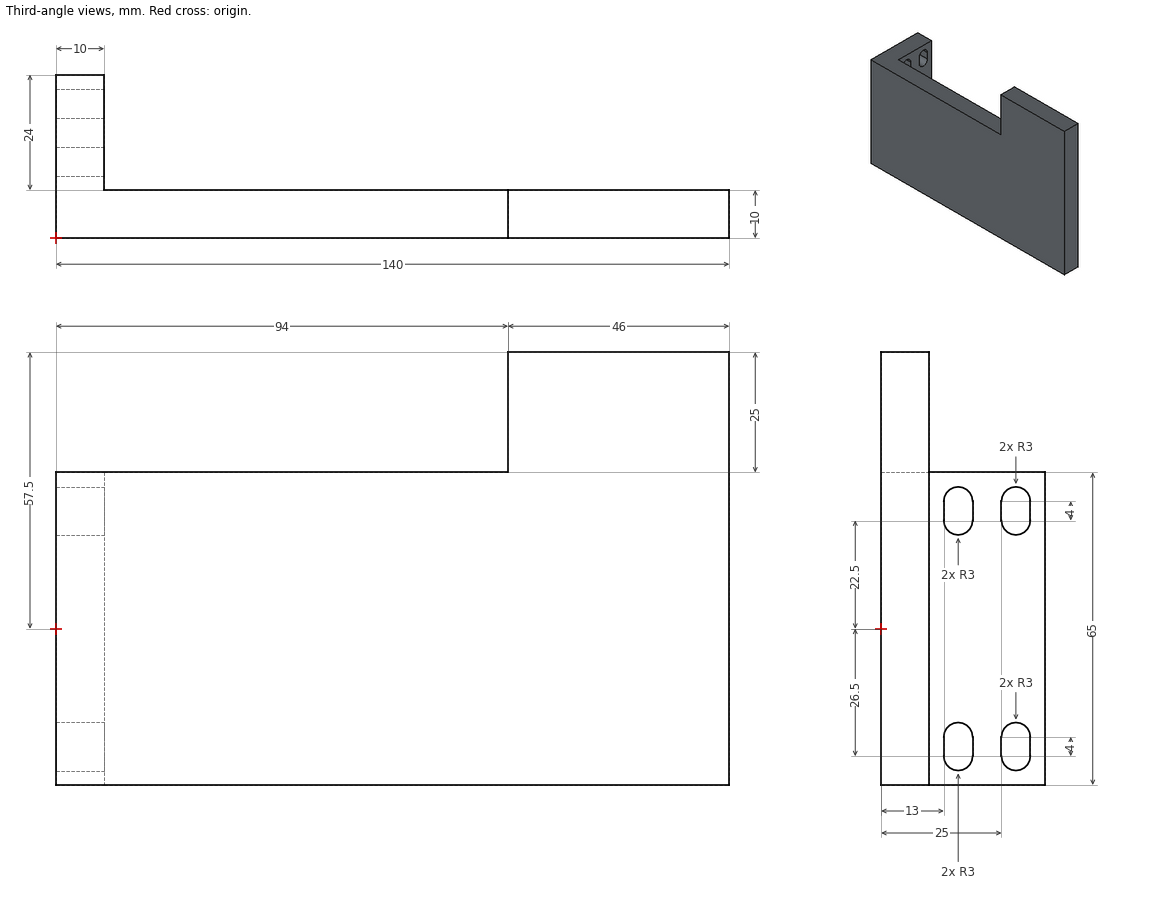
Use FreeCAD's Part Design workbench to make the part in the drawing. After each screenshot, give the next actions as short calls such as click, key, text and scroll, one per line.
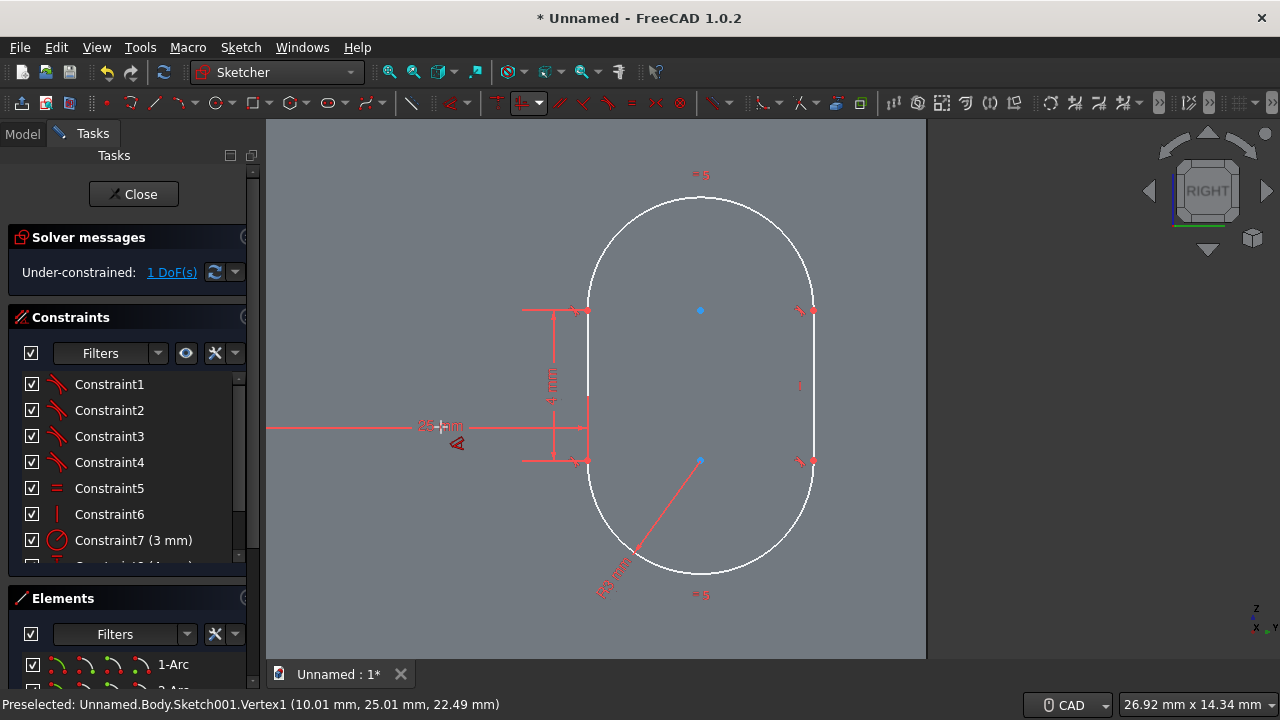
click(588, 461)
click(622, 507)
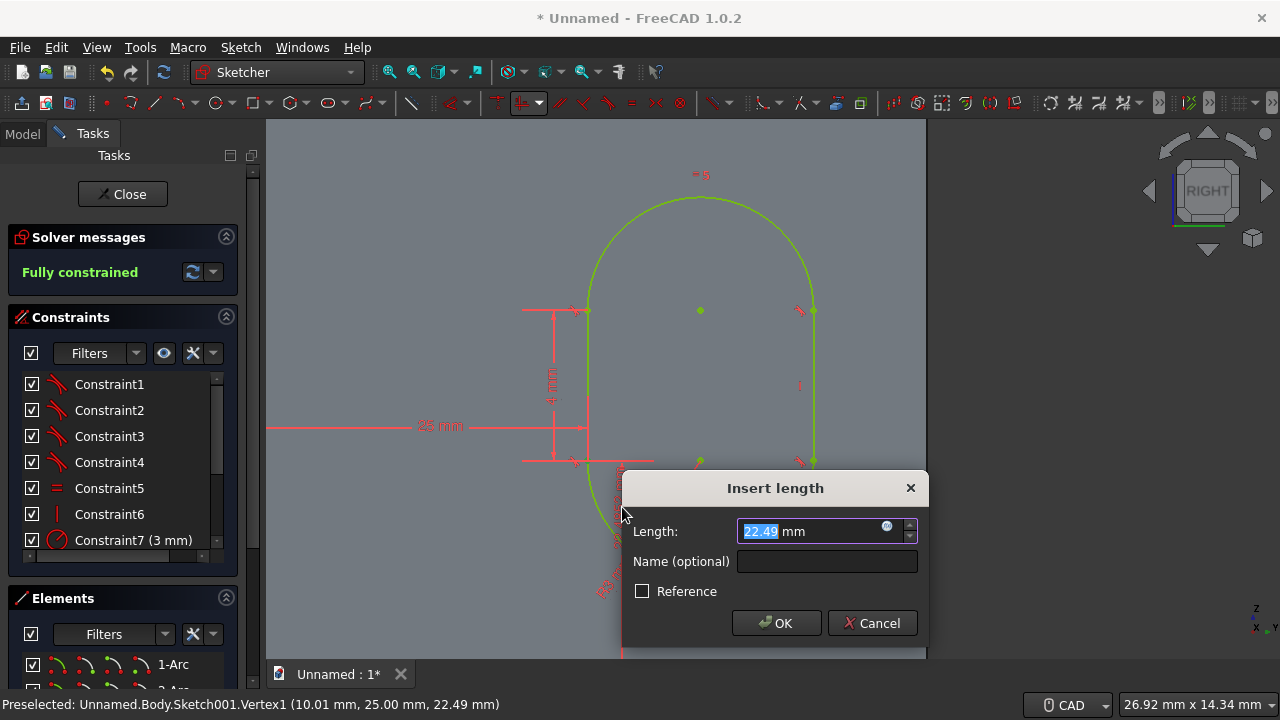
text(22.5)
key(Return)
key(Escape)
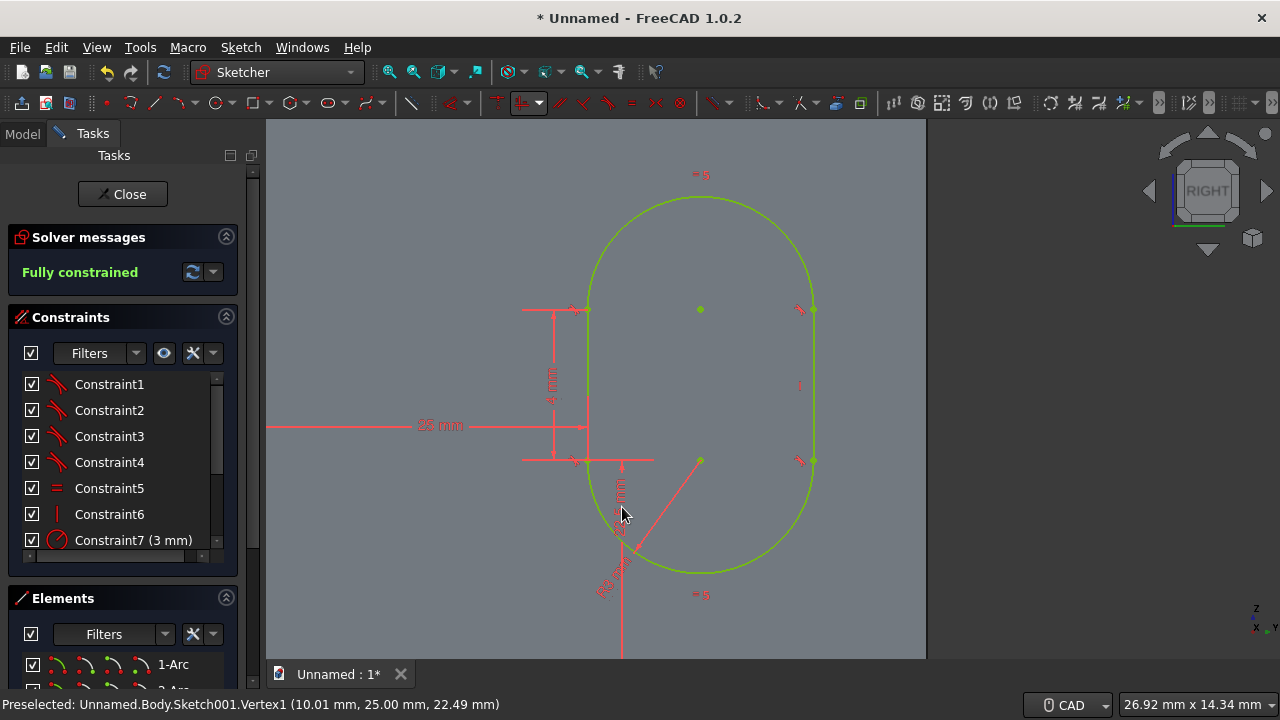
click(123, 194)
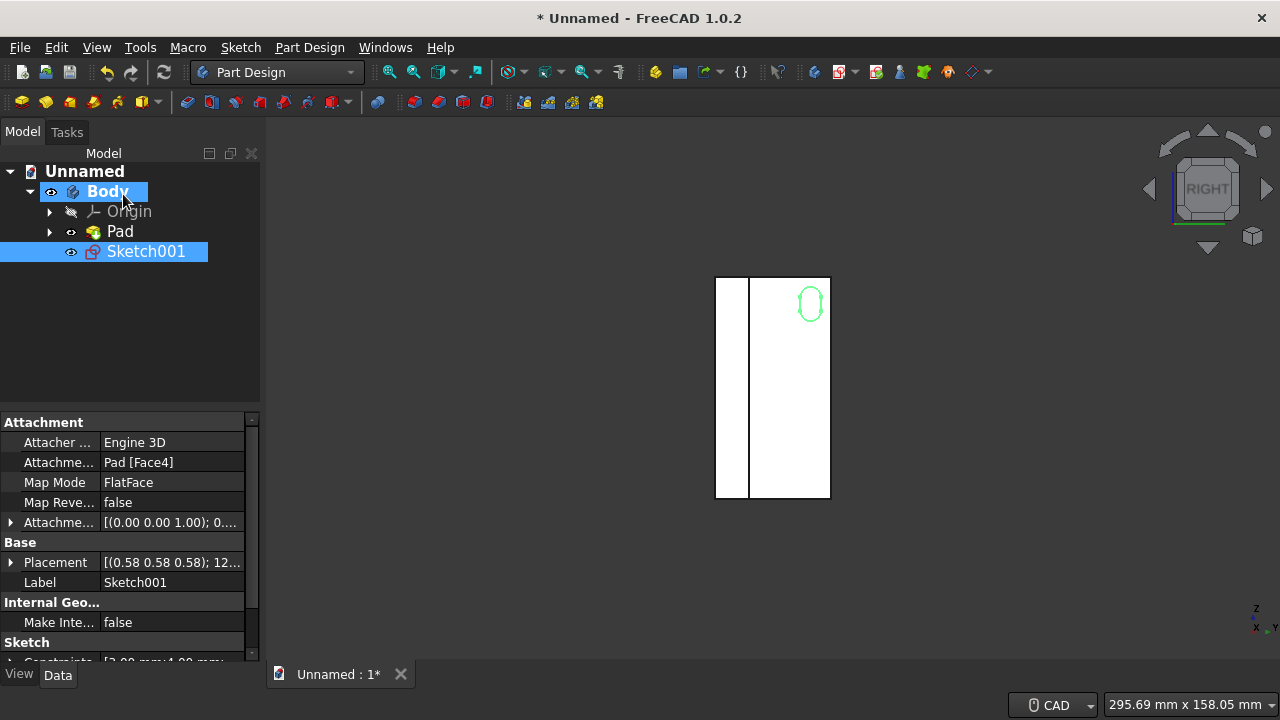
click(188, 102)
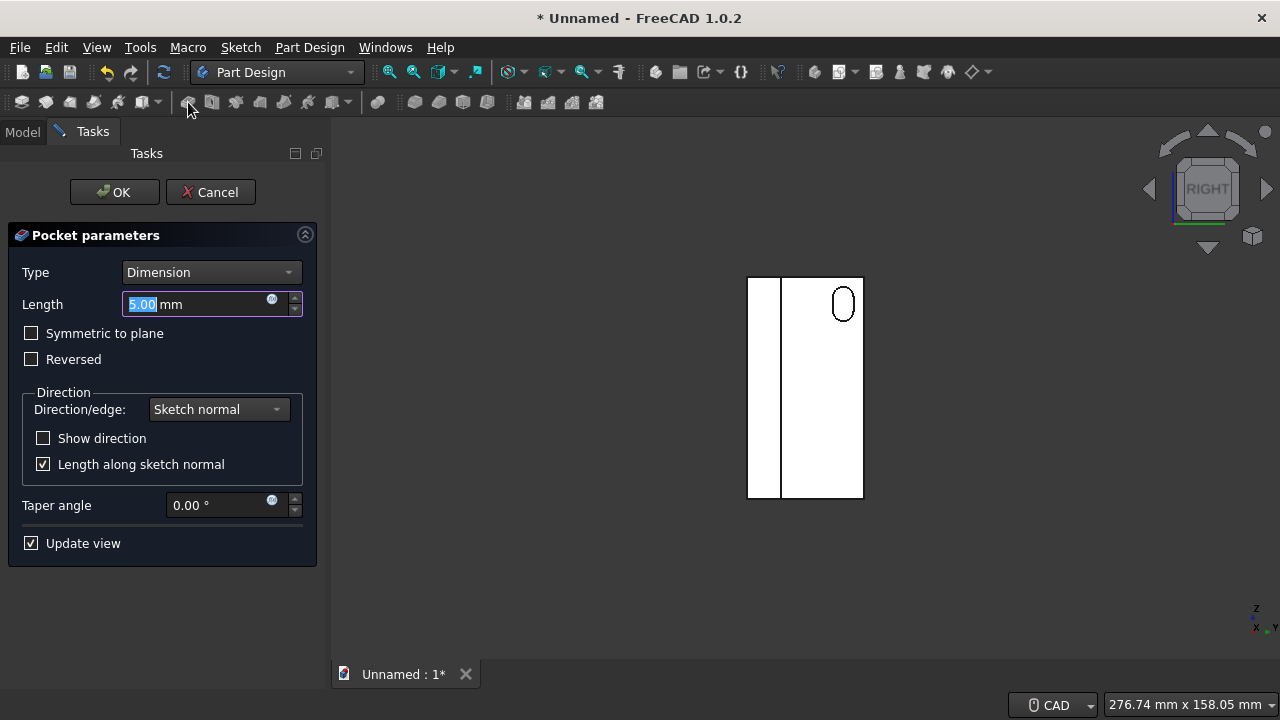
click(212, 272)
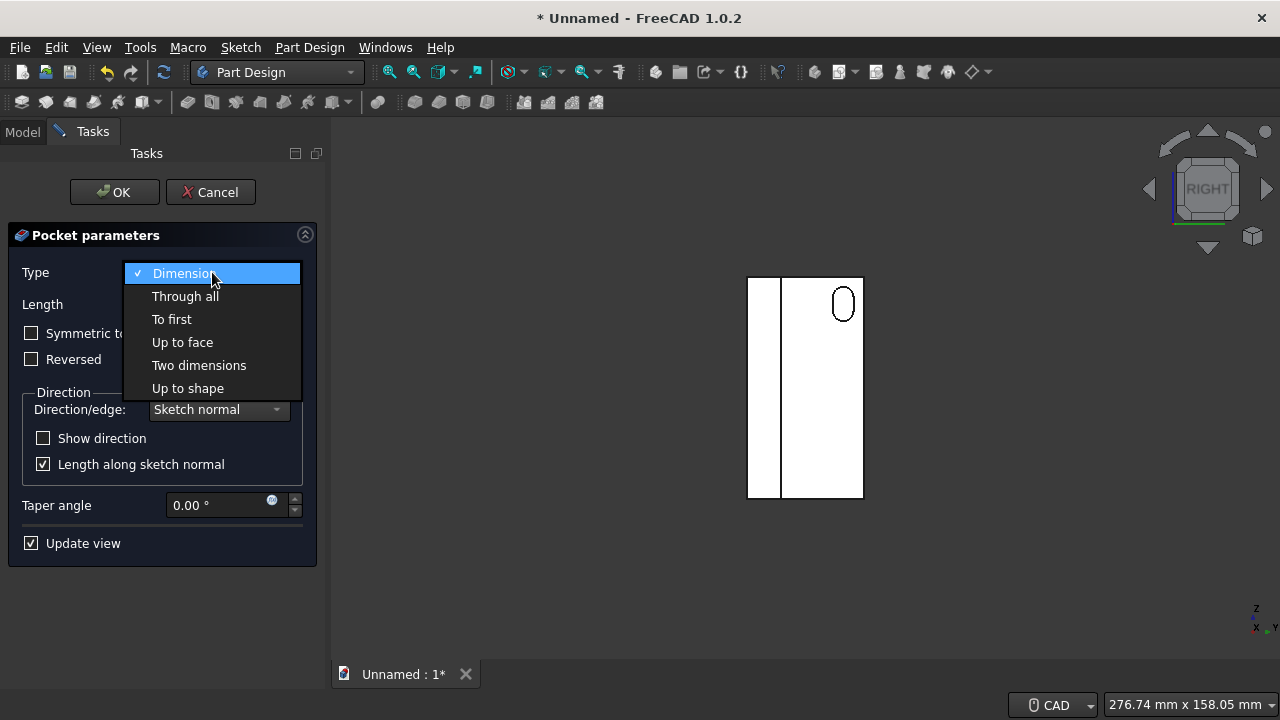
click(212, 320)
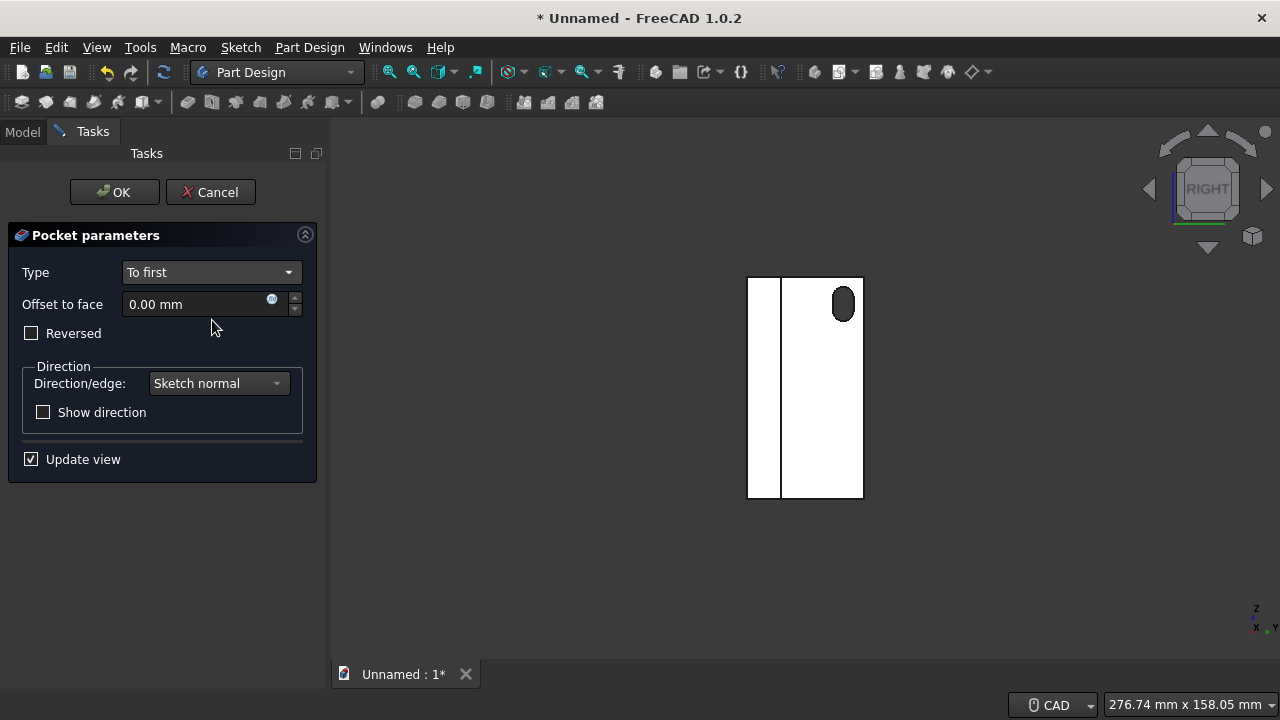
click(115, 192)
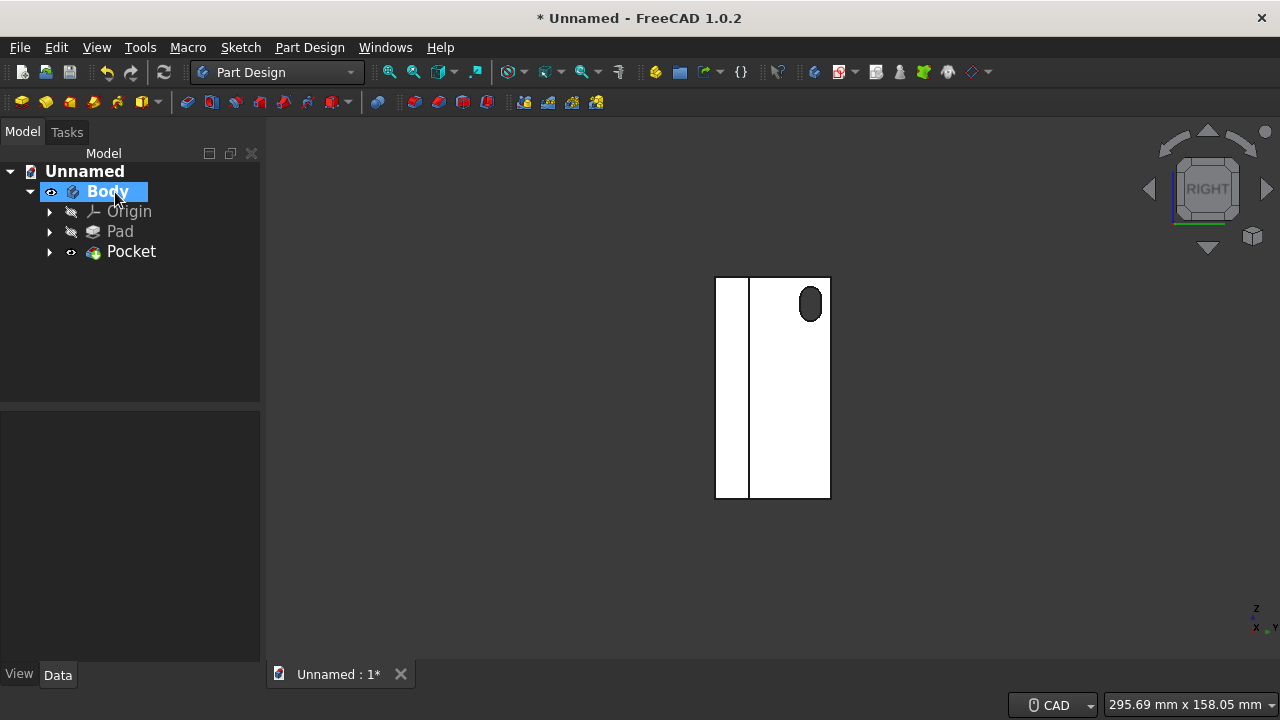
key(v)
key(f)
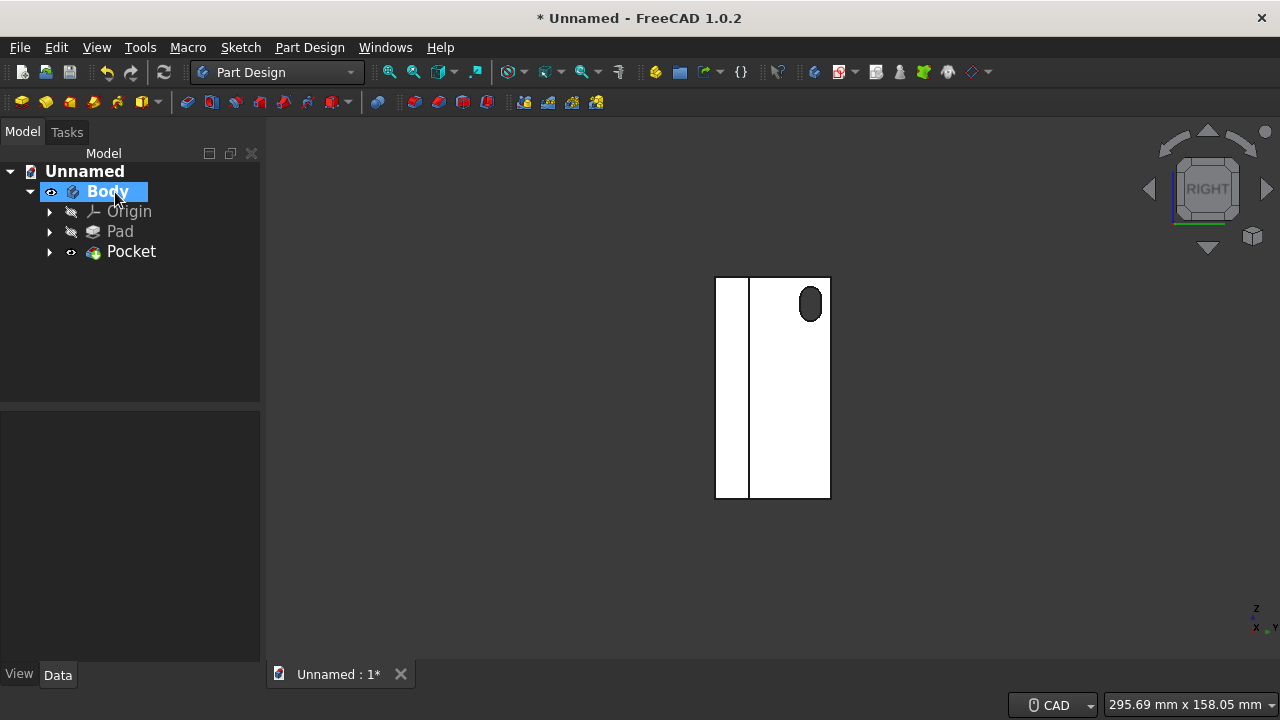
click(790, 387)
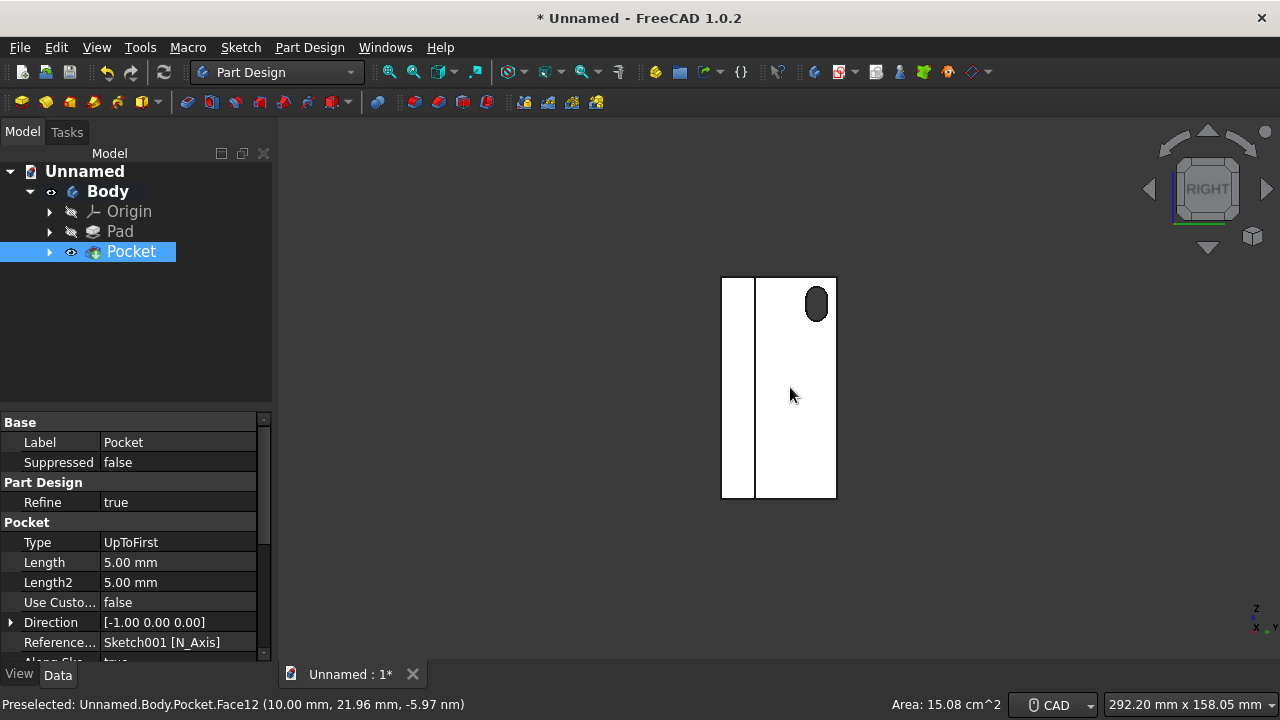
click(840, 72)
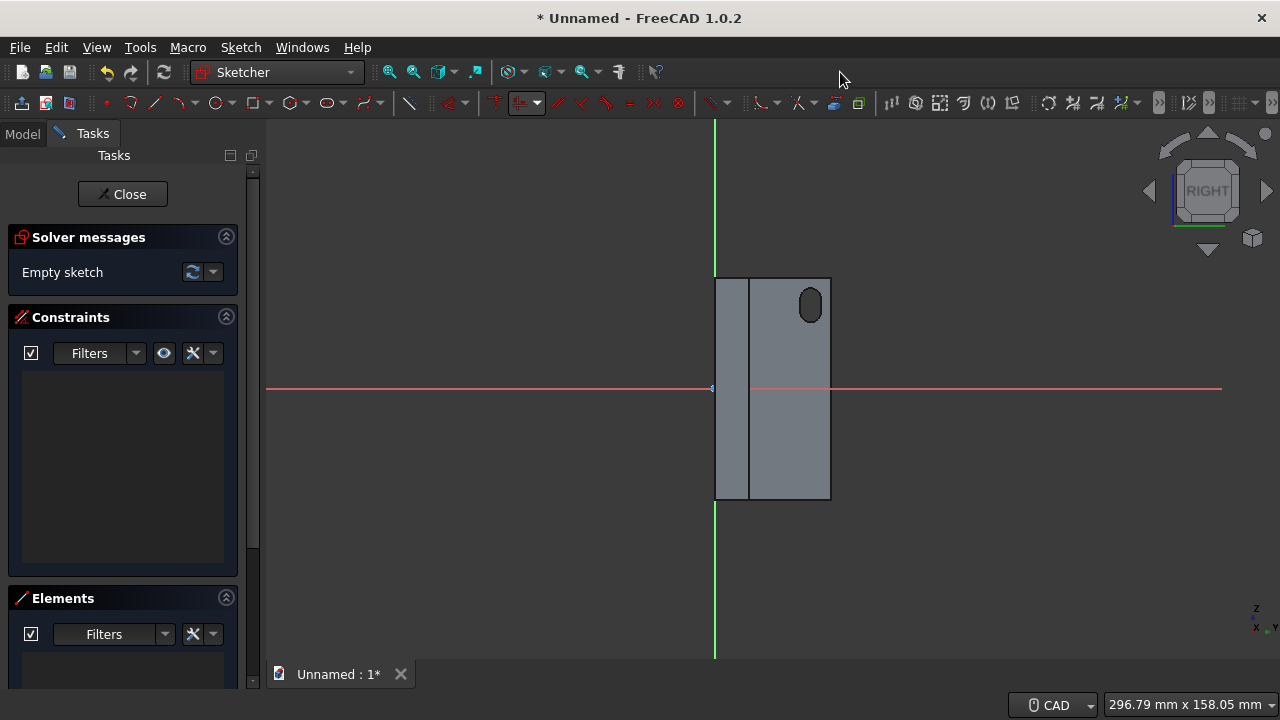
scroll(821, 481, up, 12)